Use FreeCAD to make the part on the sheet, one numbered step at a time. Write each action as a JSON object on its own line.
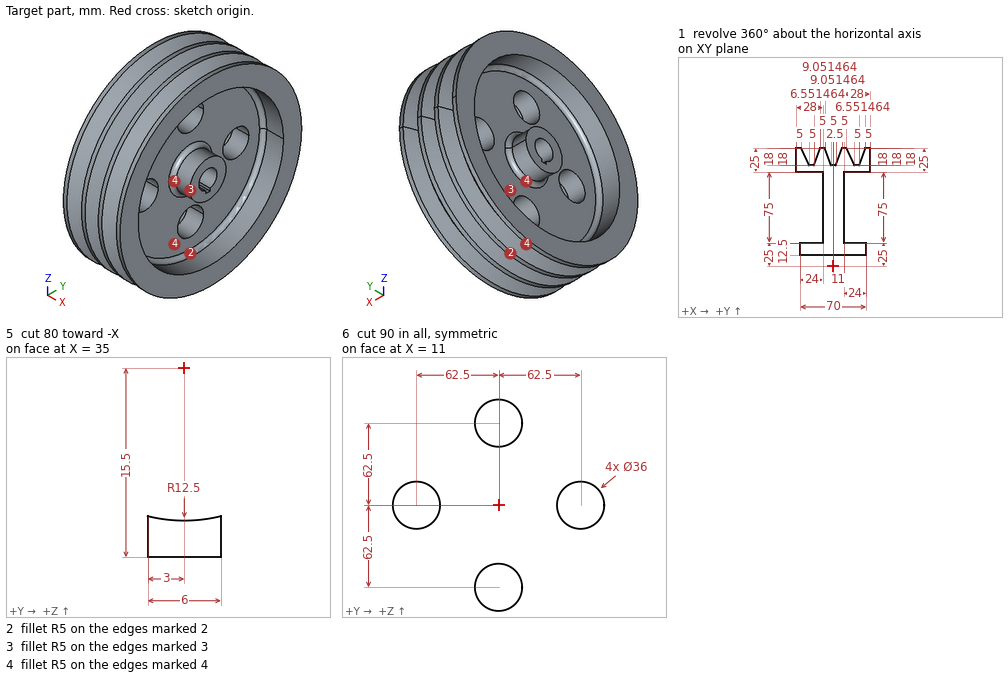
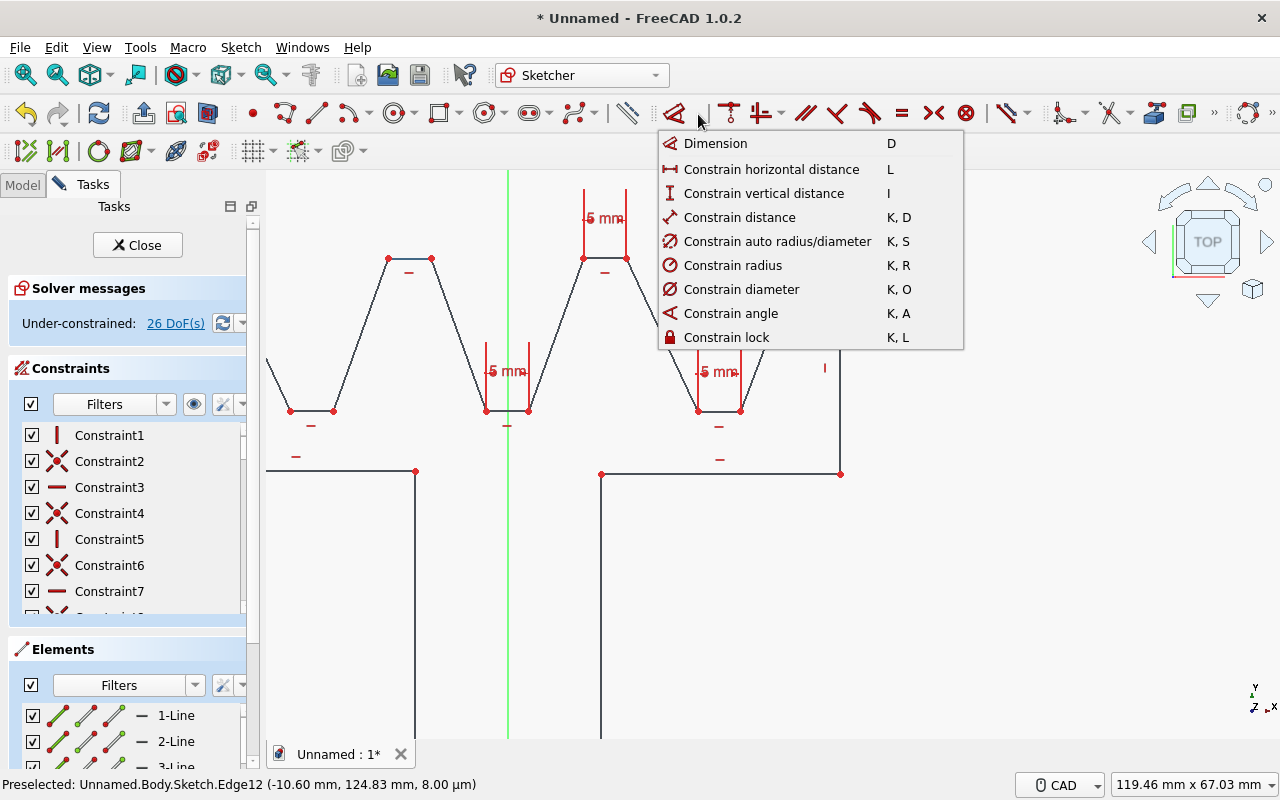
{"action": "left_click", "coordinate": [811, 169]}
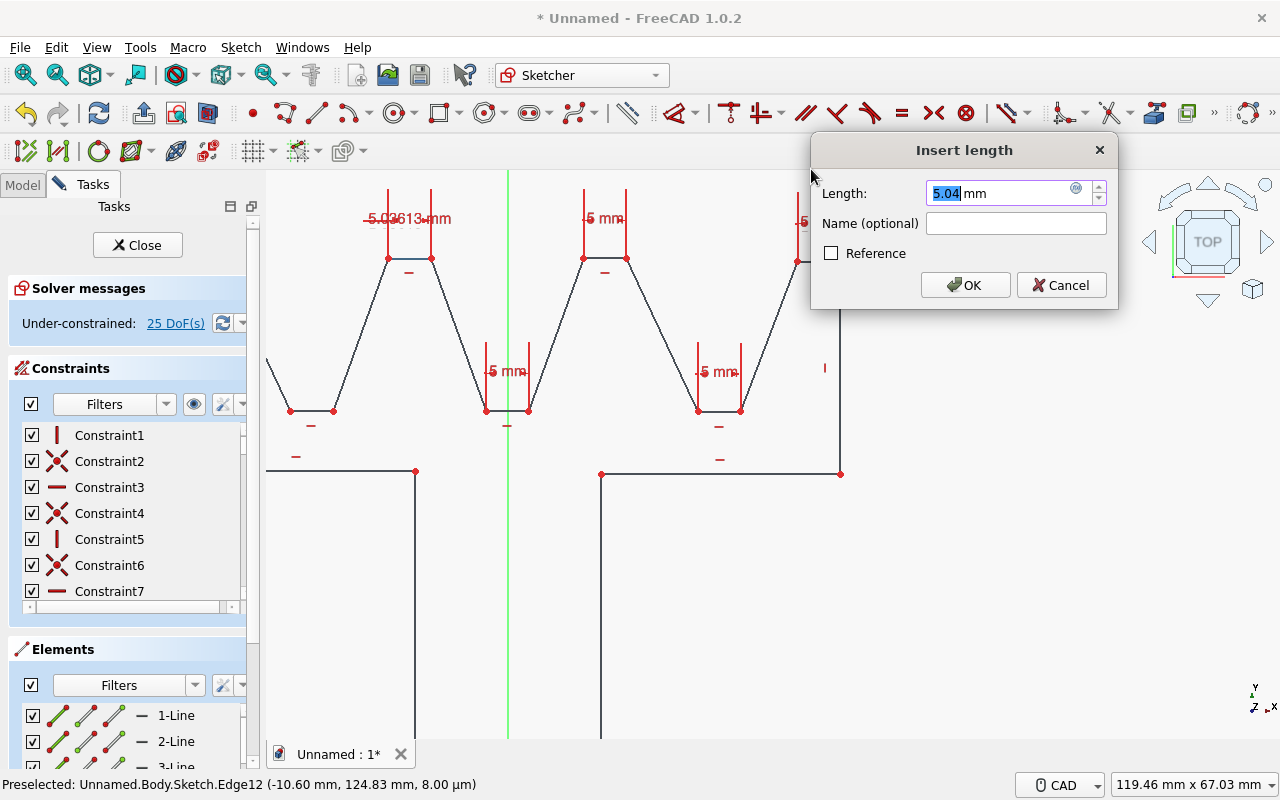
{"action": "type", "text": "5"}
{"action": "key", "text": "Return"}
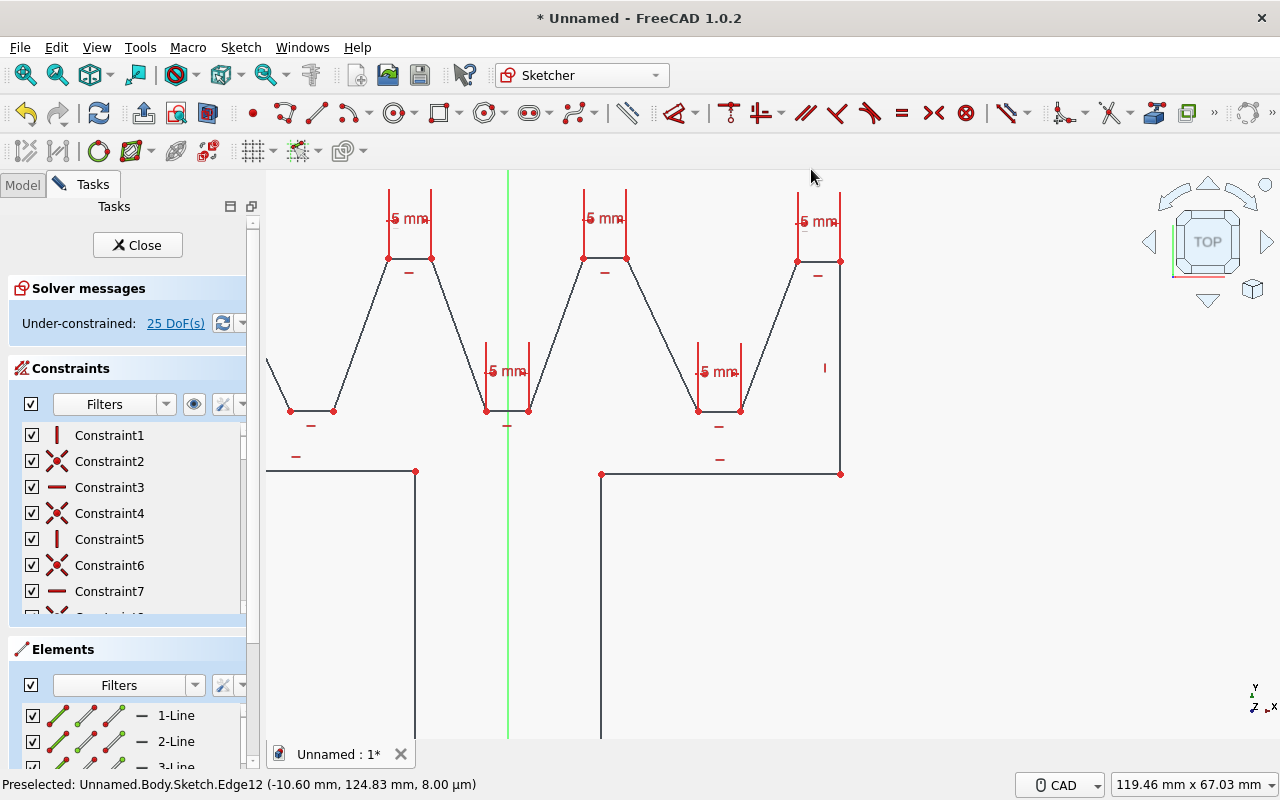
{"action": "left_click", "coordinate": [320, 411]}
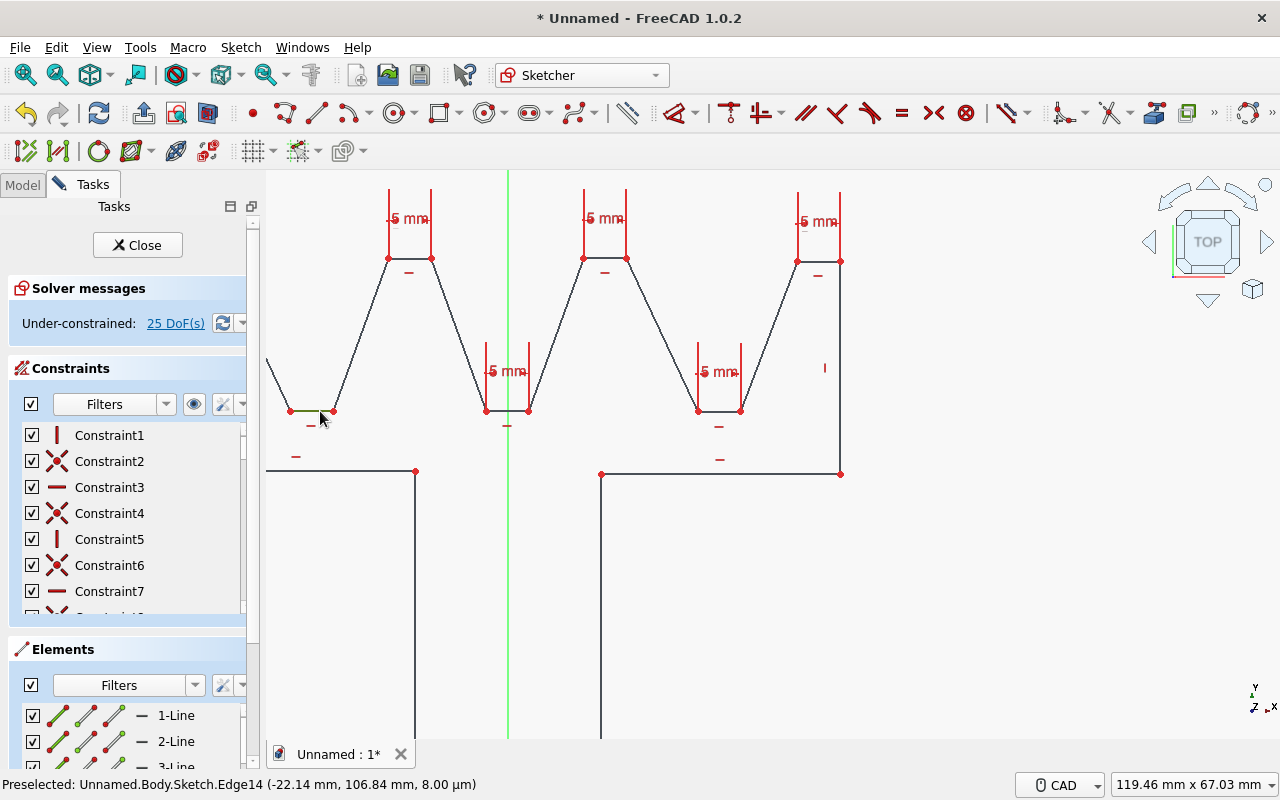
{"action": "key", "text": "l"}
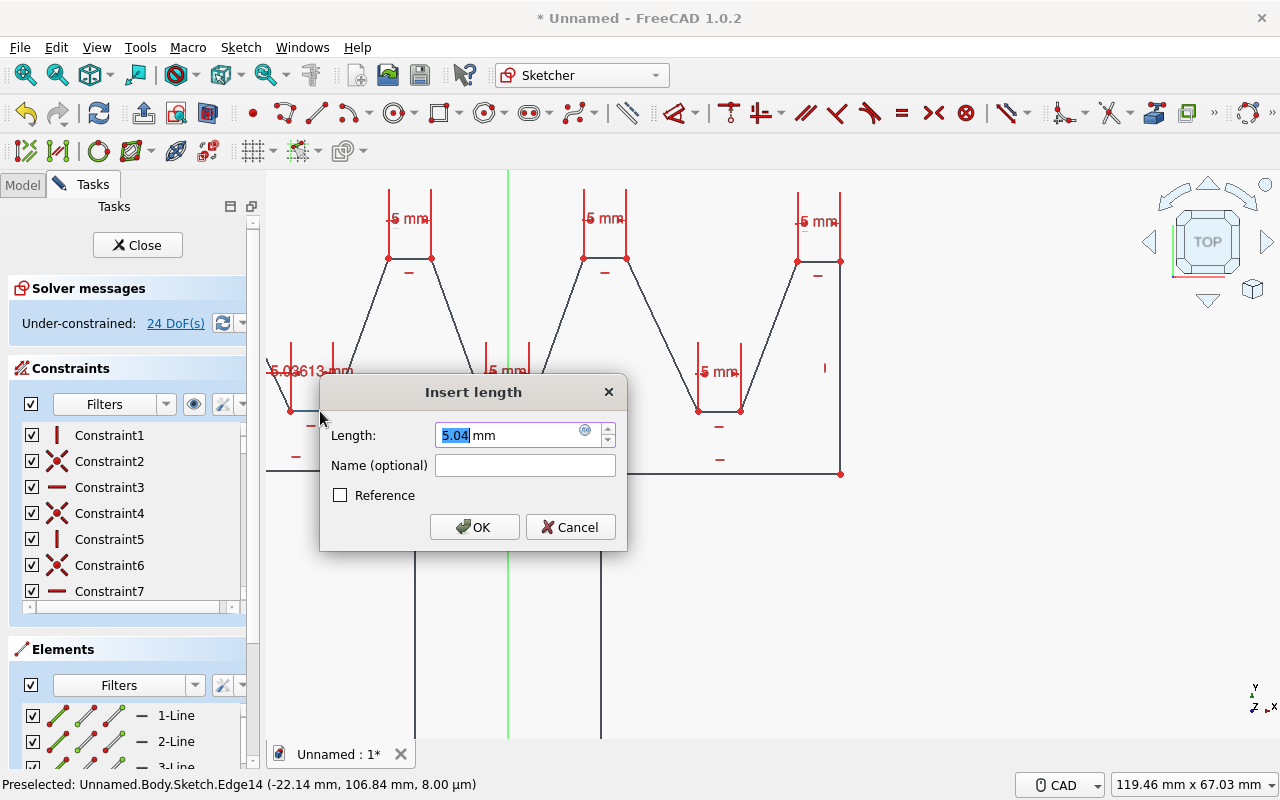
{"action": "type", "text": "5"}
{"action": "key", "text": "Return"}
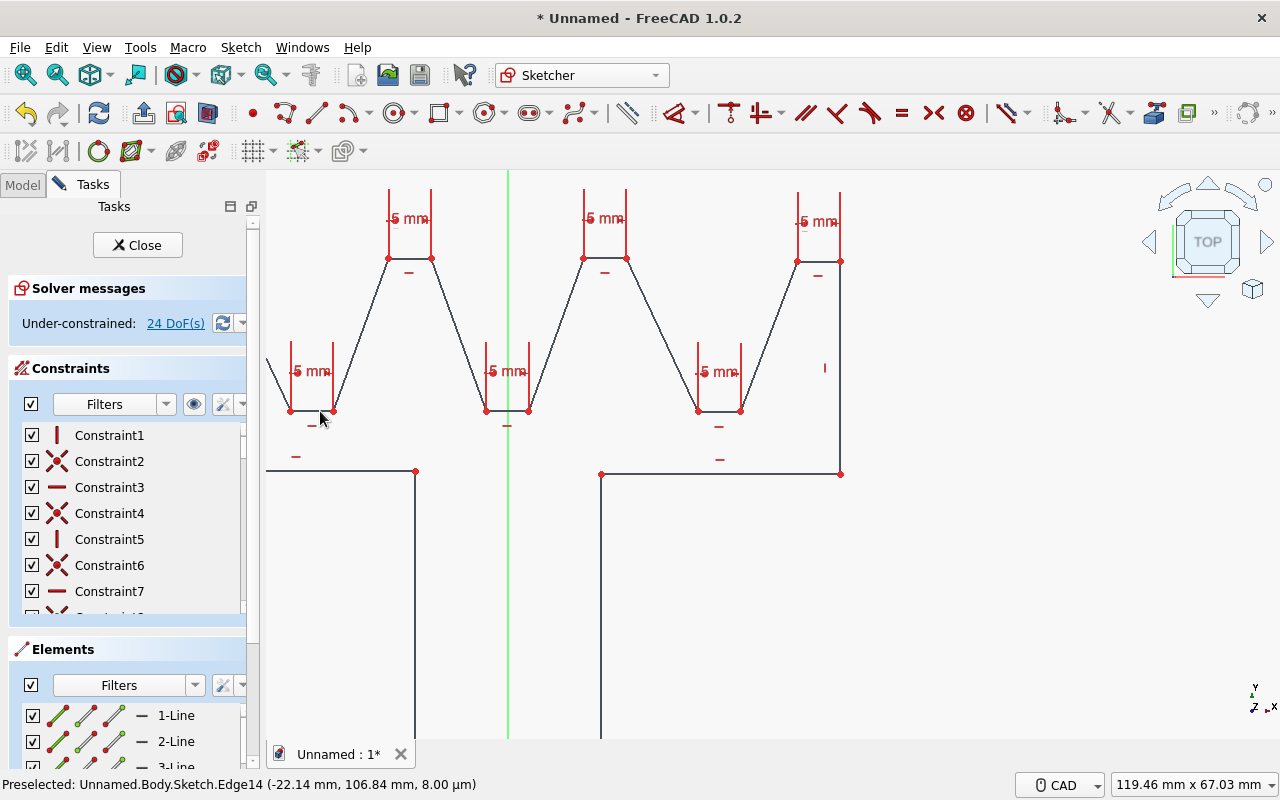
{"action": "scroll", "coordinate": [819, 261], "scroll_direction": "down", "scroll_amount": 5}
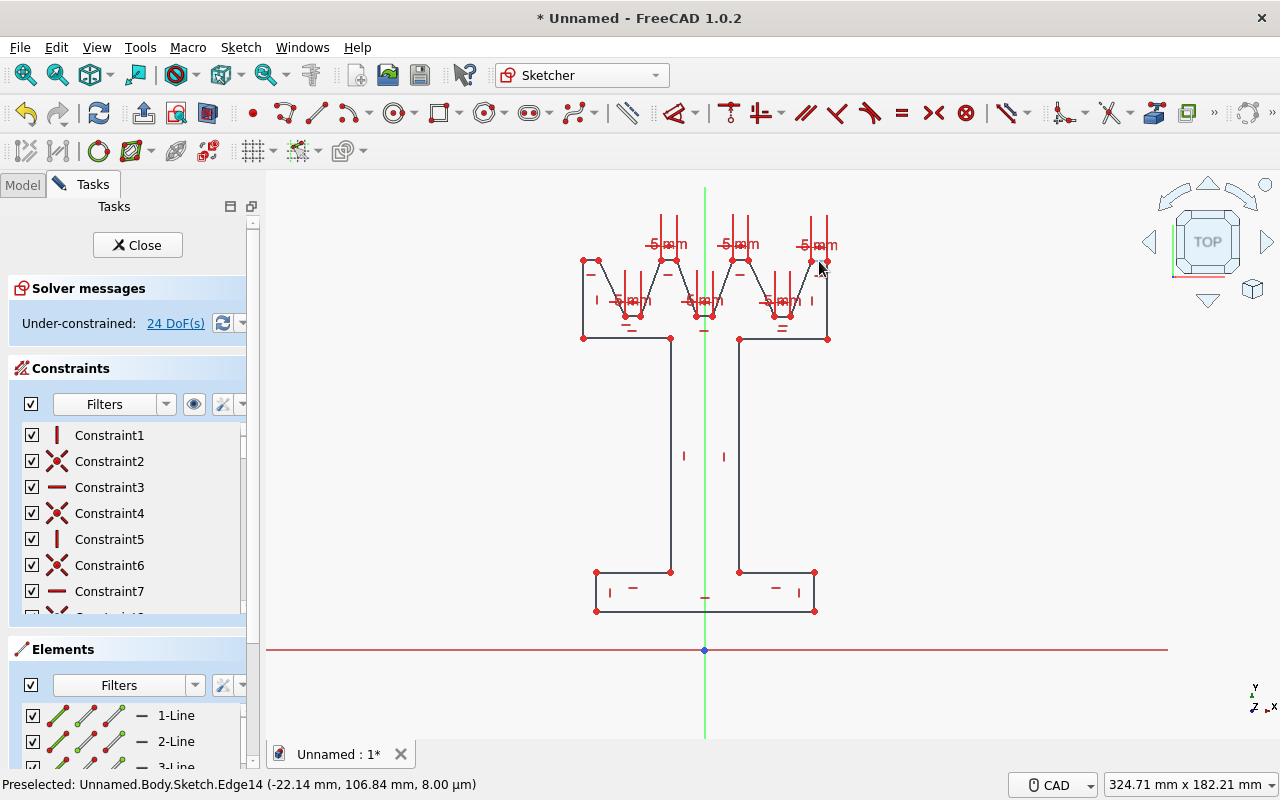
{"action": "scroll", "coordinate": [594, 260], "scroll_direction": "up", "scroll_amount": 6}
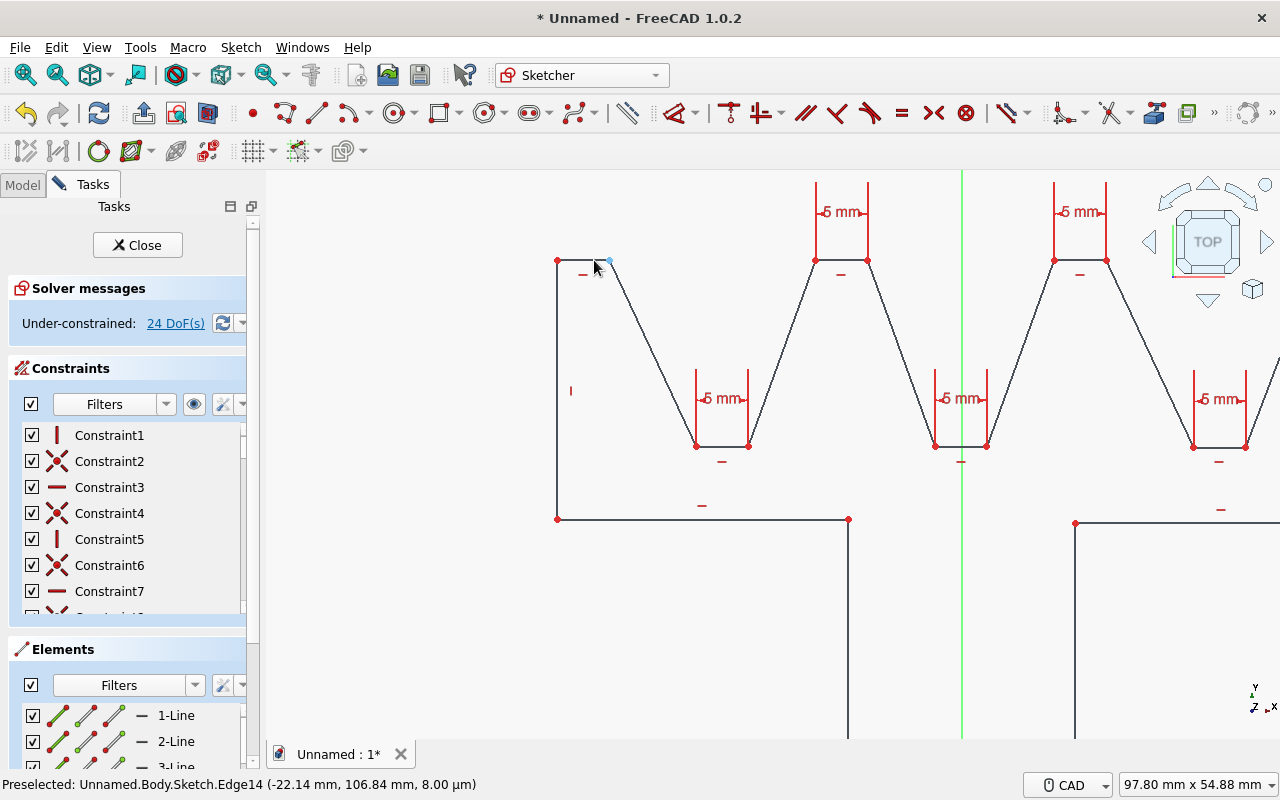
{"action": "left_click", "coordinate": [594, 260]}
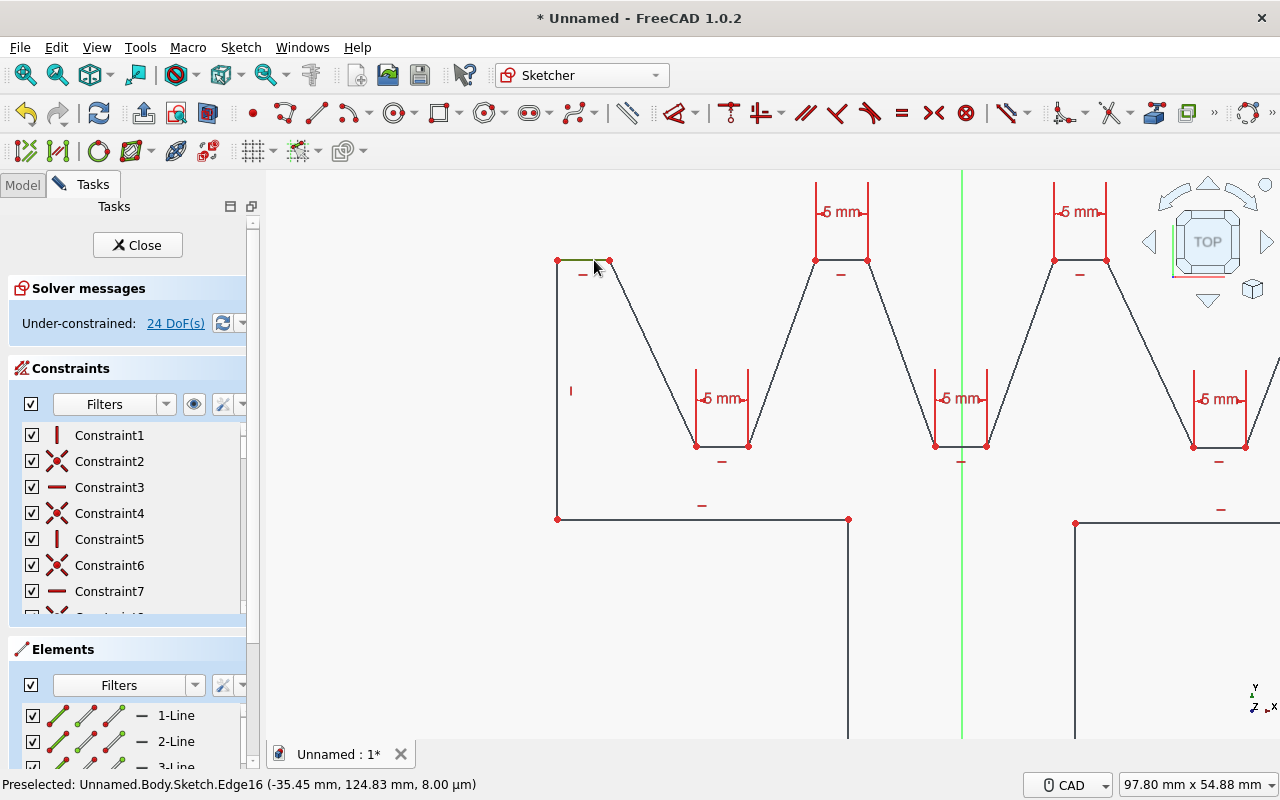
{"action": "key", "text": "l"}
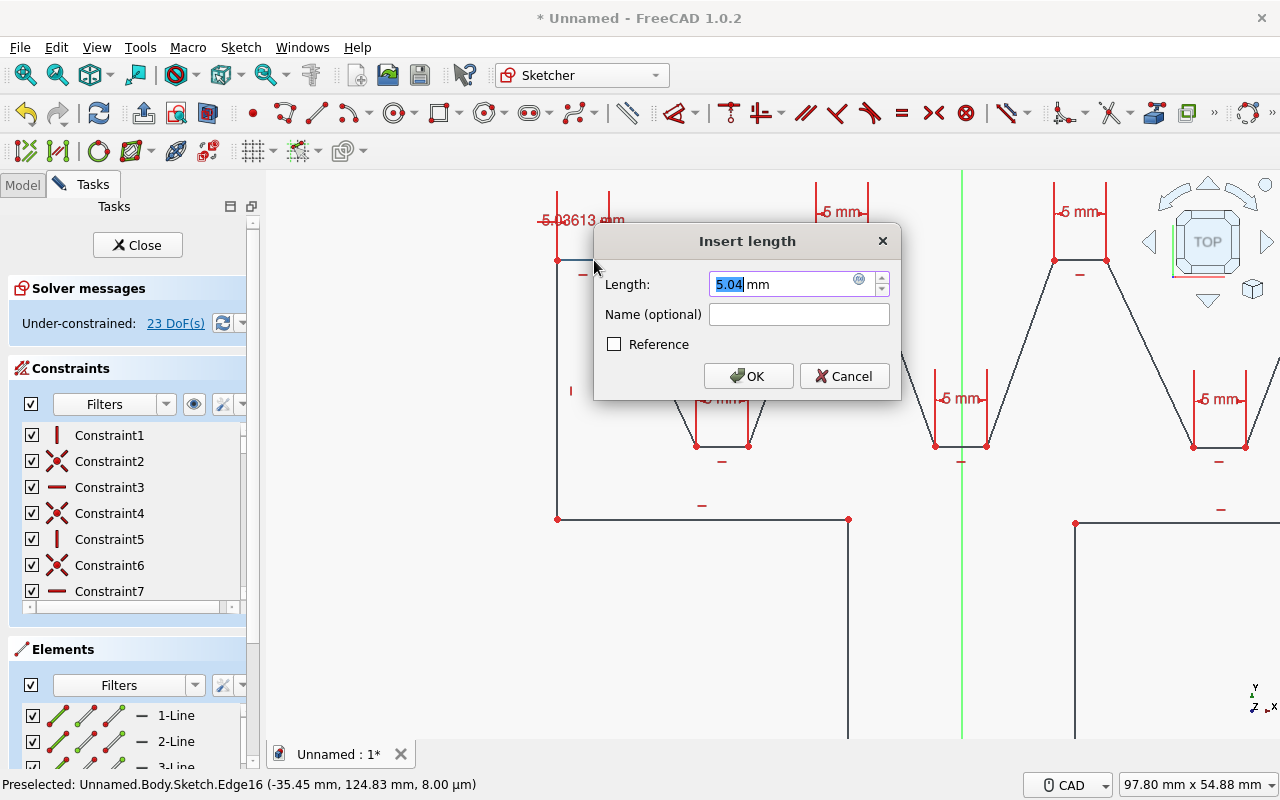
{"action": "type", "text": "5"}
{"action": "key", "text": "Return"}